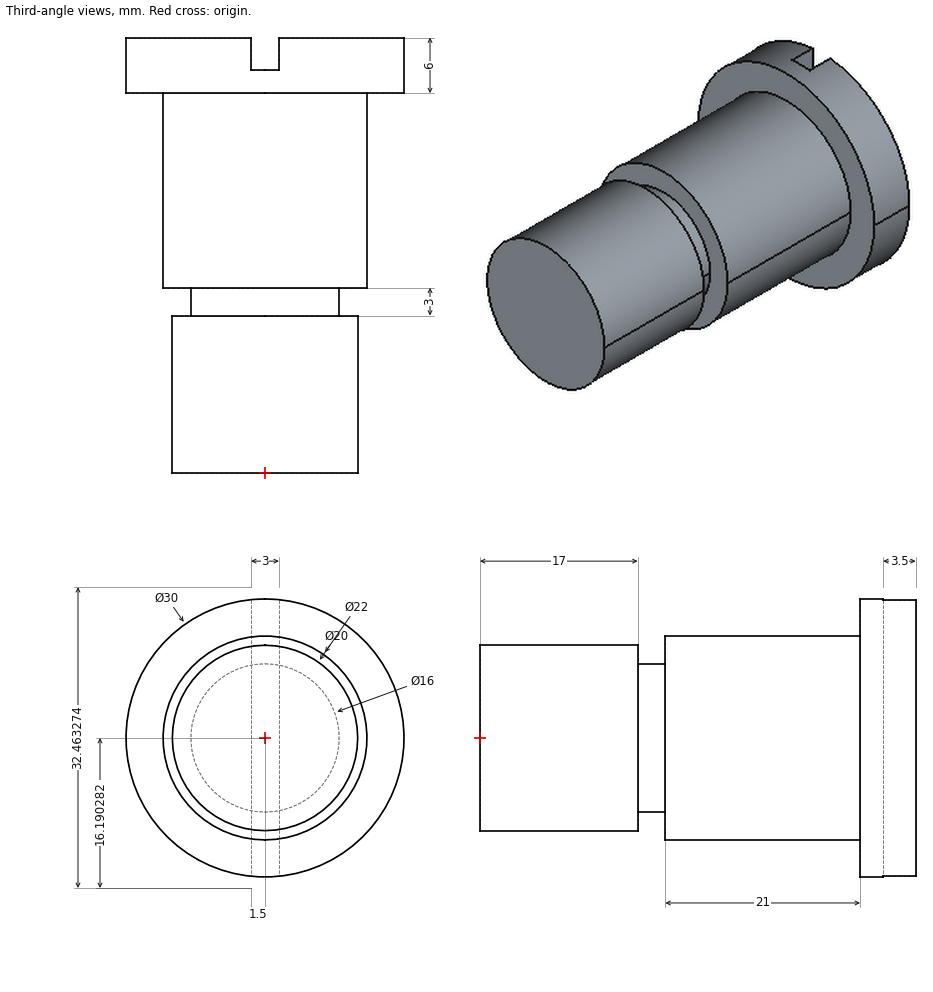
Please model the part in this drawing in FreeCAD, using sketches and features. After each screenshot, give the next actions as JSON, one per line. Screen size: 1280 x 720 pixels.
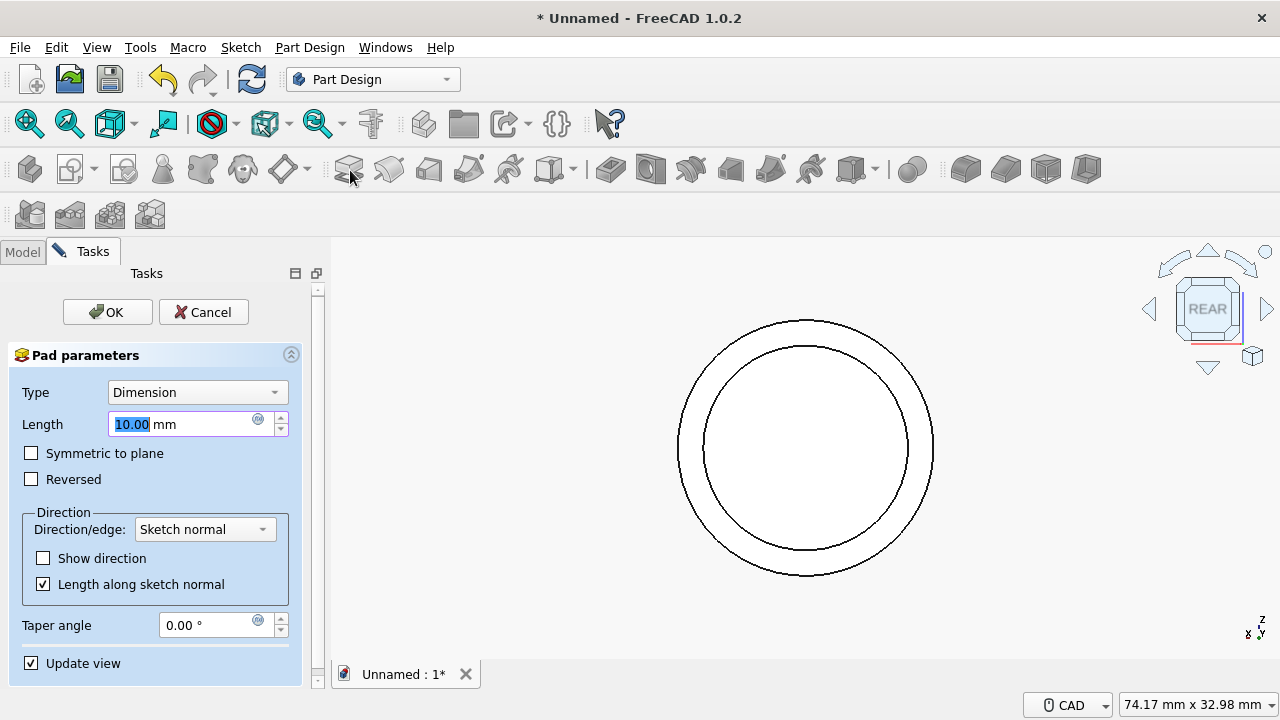
{"action": "type", "text": "3"}
{"action": "key", "text": "Tab"}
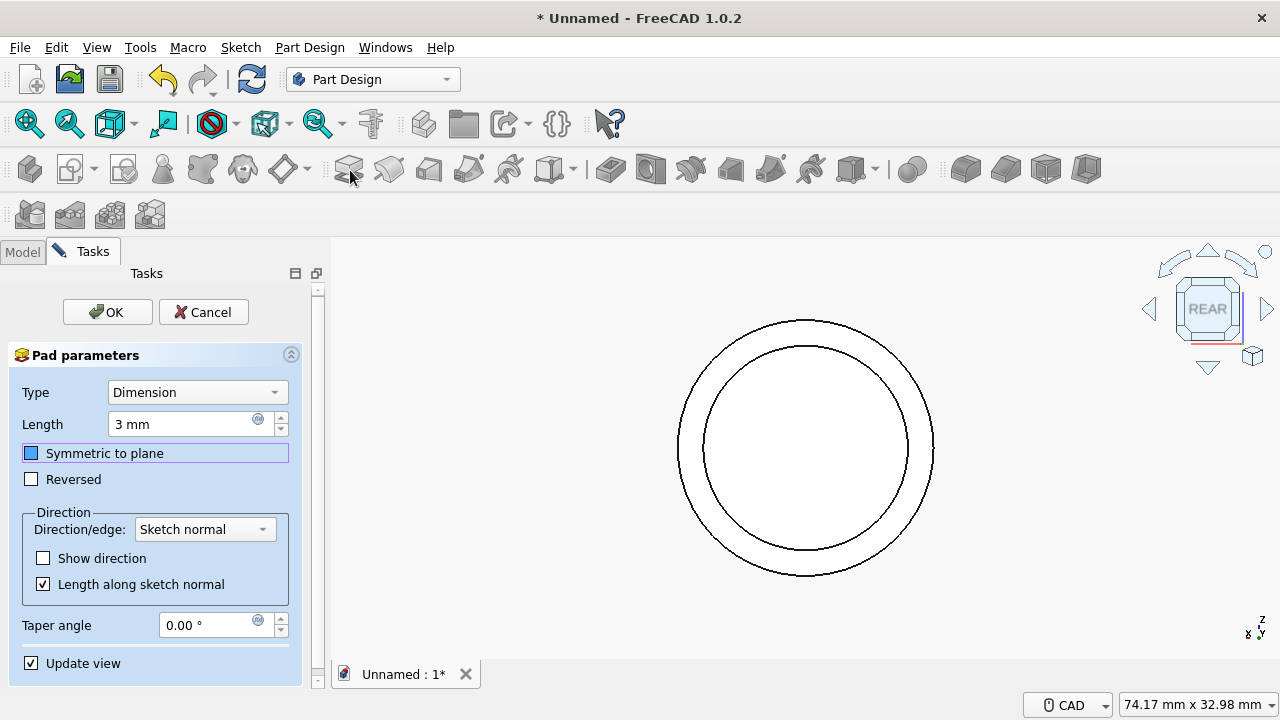
{"action": "left_click", "coordinate": [108, 312]}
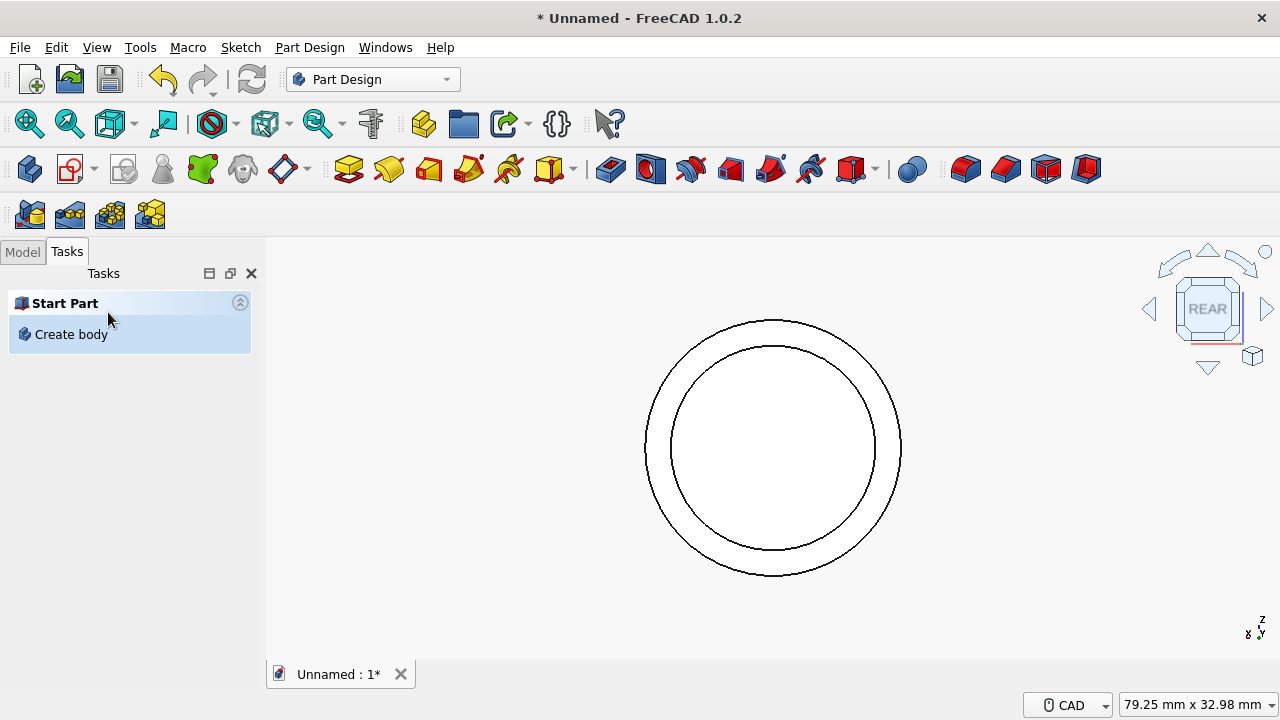
{"action": "left_click", "coordinate": [773, 447]}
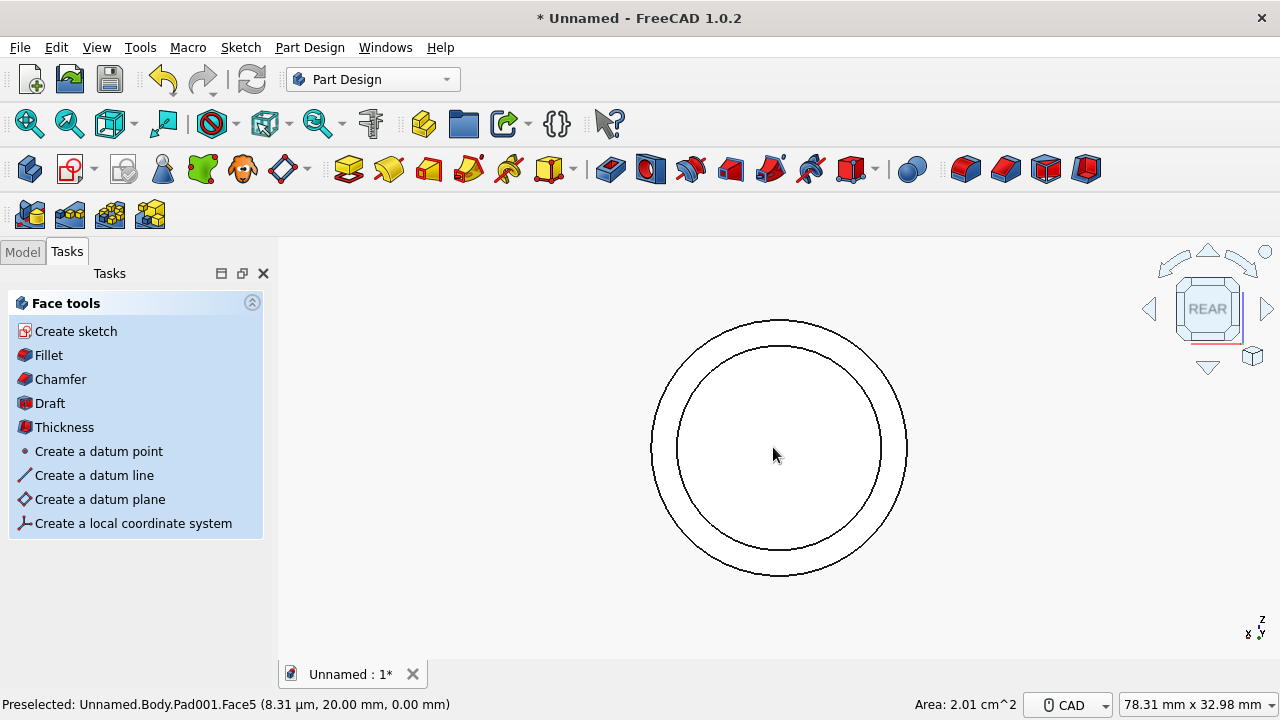
{"action": "left_click", "coordinate": [70, 170]}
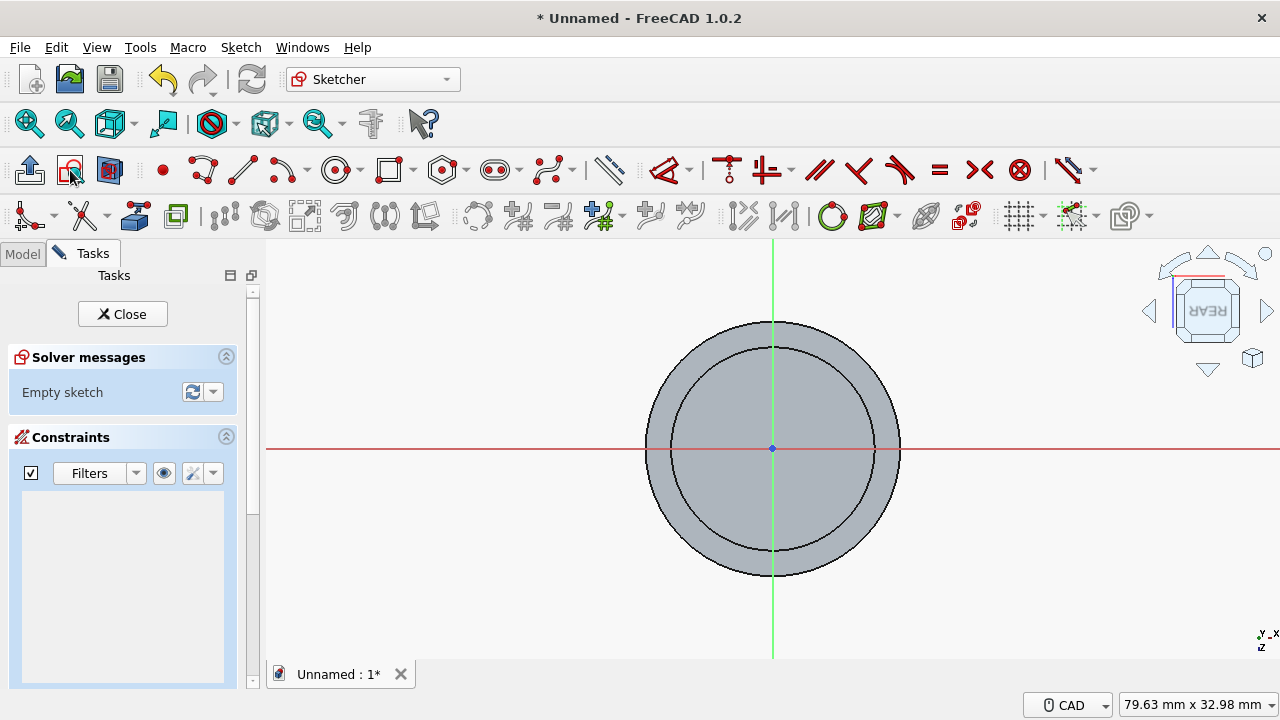
{"action": "left_click", "coordinate": [336, 170]}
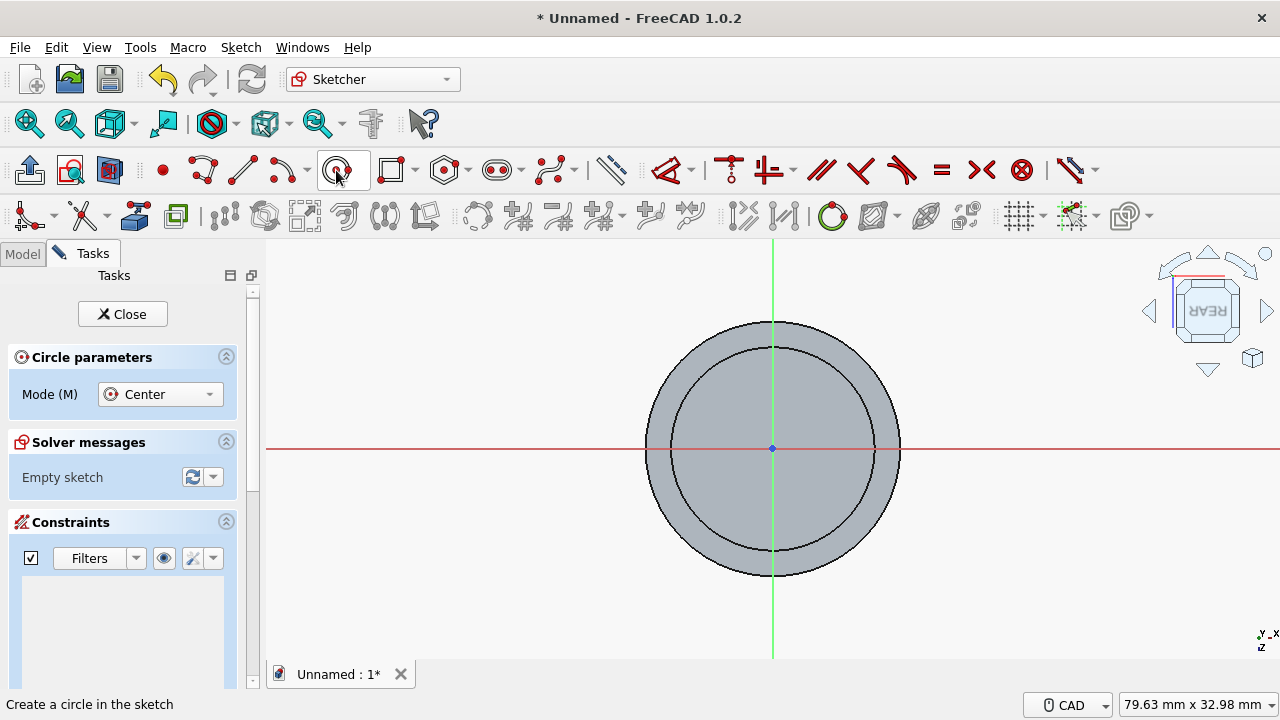
{"action": "left_click", "coordinate": [773, 449]}
{"action": "mouse_move", "coordinate": [872, 350]}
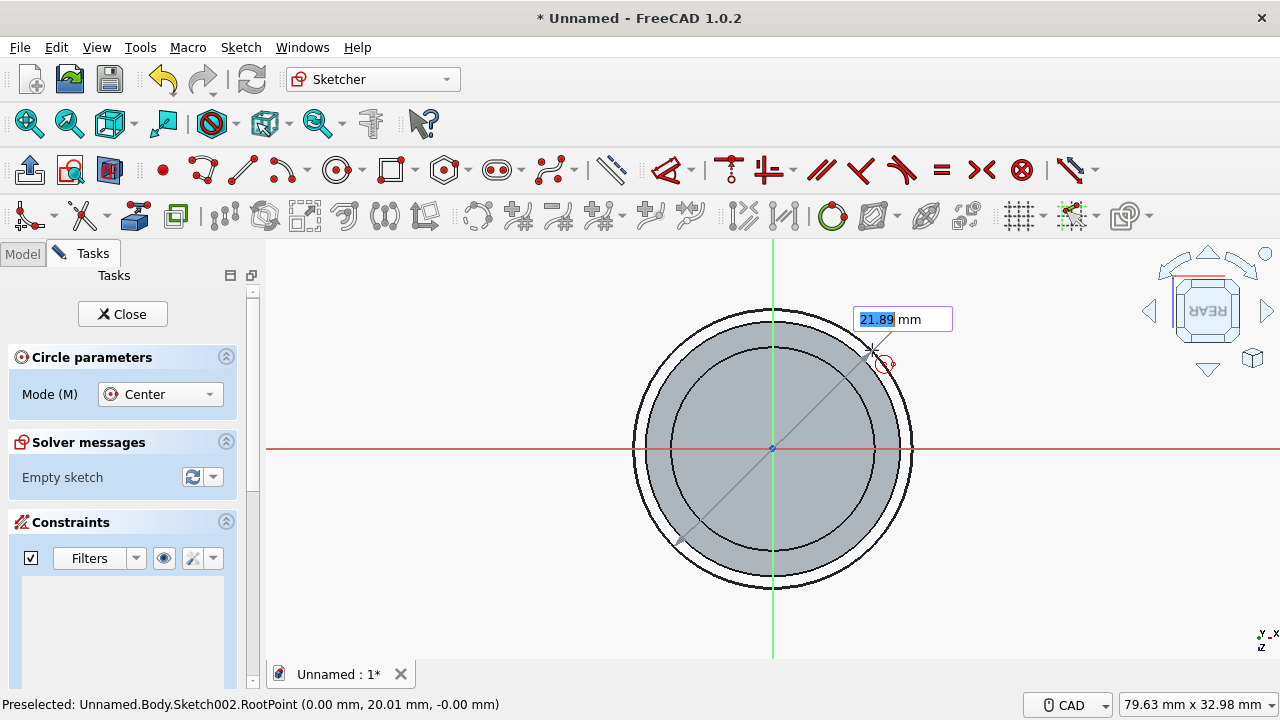
{"action": "type", "text": "22"}
{"action": "key", "text": "Return"}
{"action": "key", "text": "Escape"}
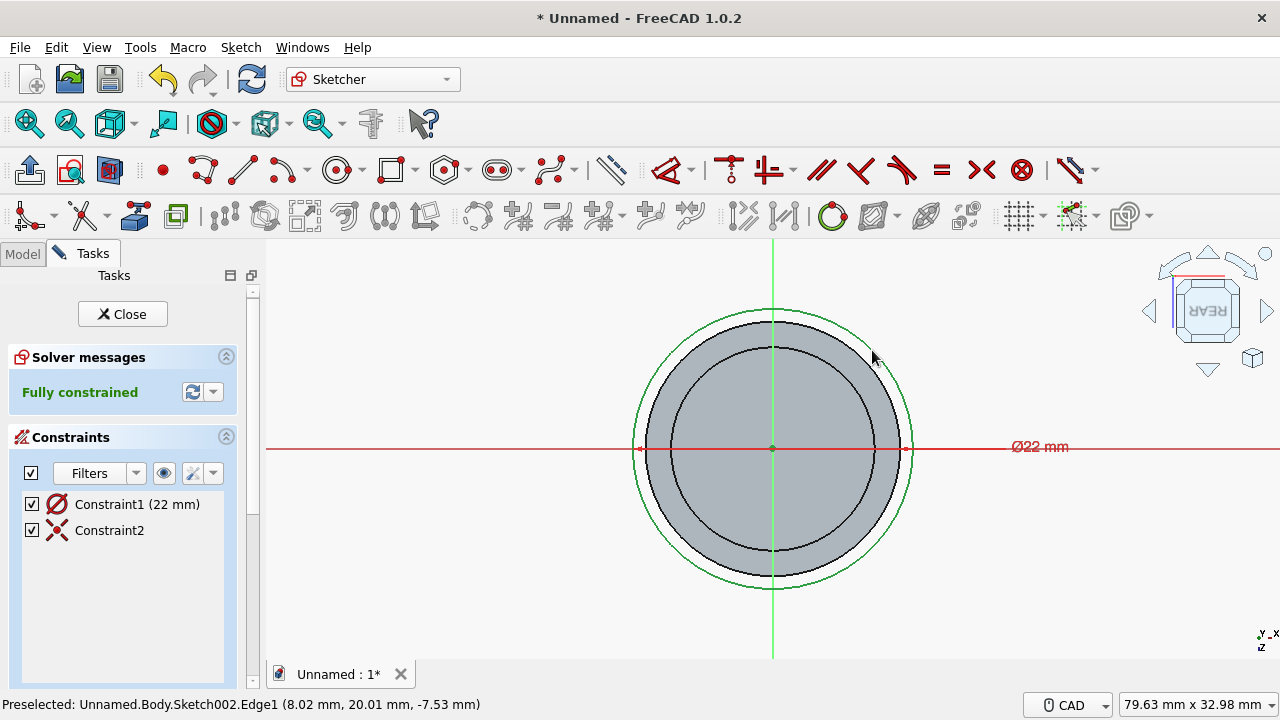
{"action": "left_click", "coordinate": [123, 314]}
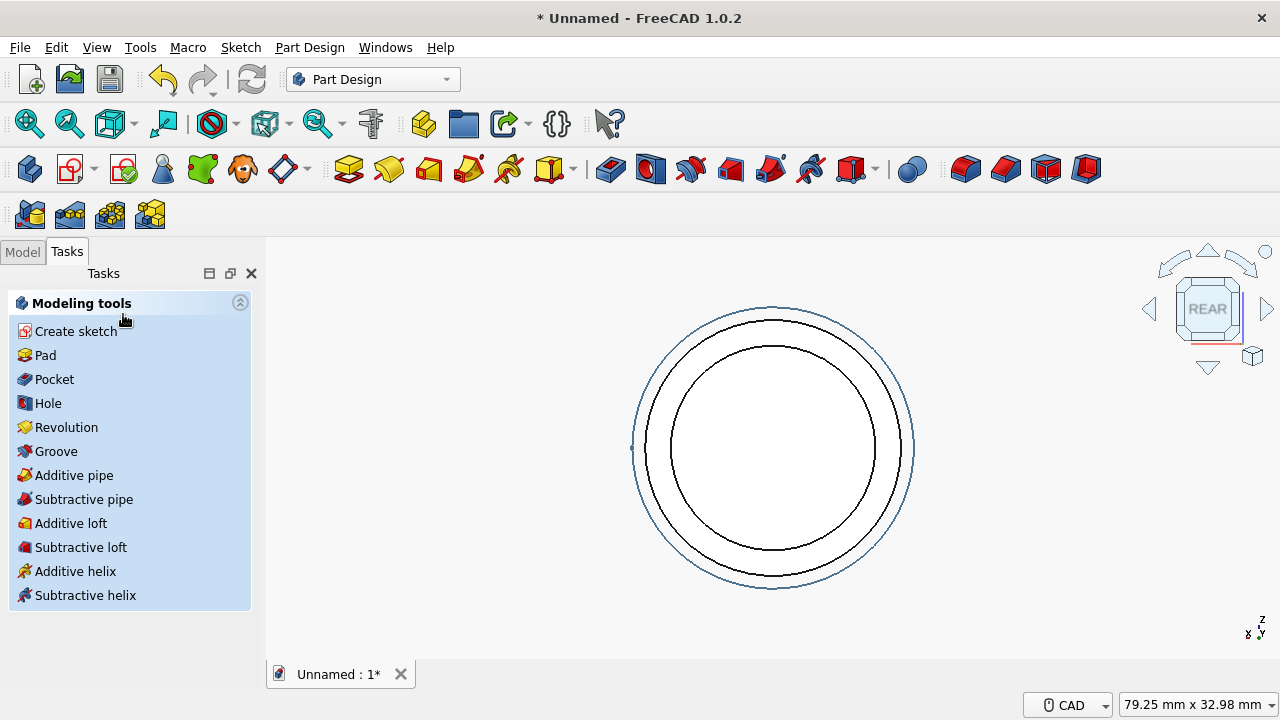
{"action": "left_click", "coordinate": [350, 170]}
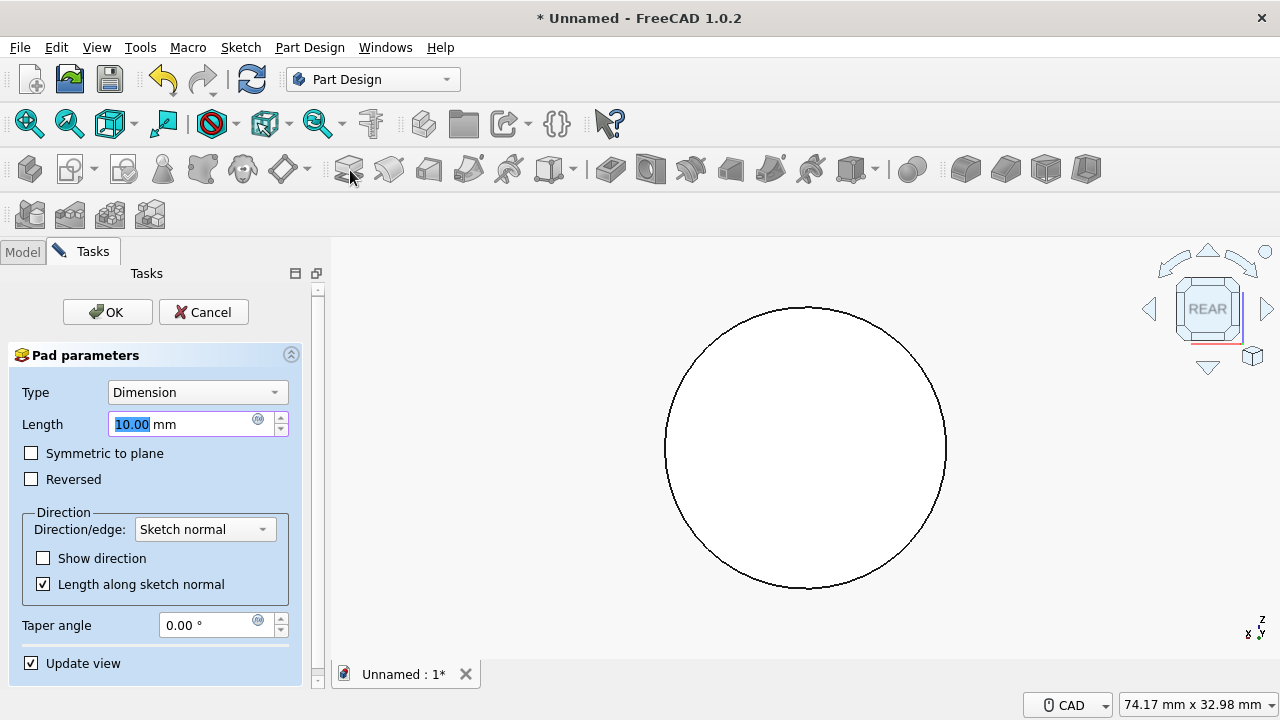
{"action": "type", "text": "21"}
{"action": "key", "text": "Tab"}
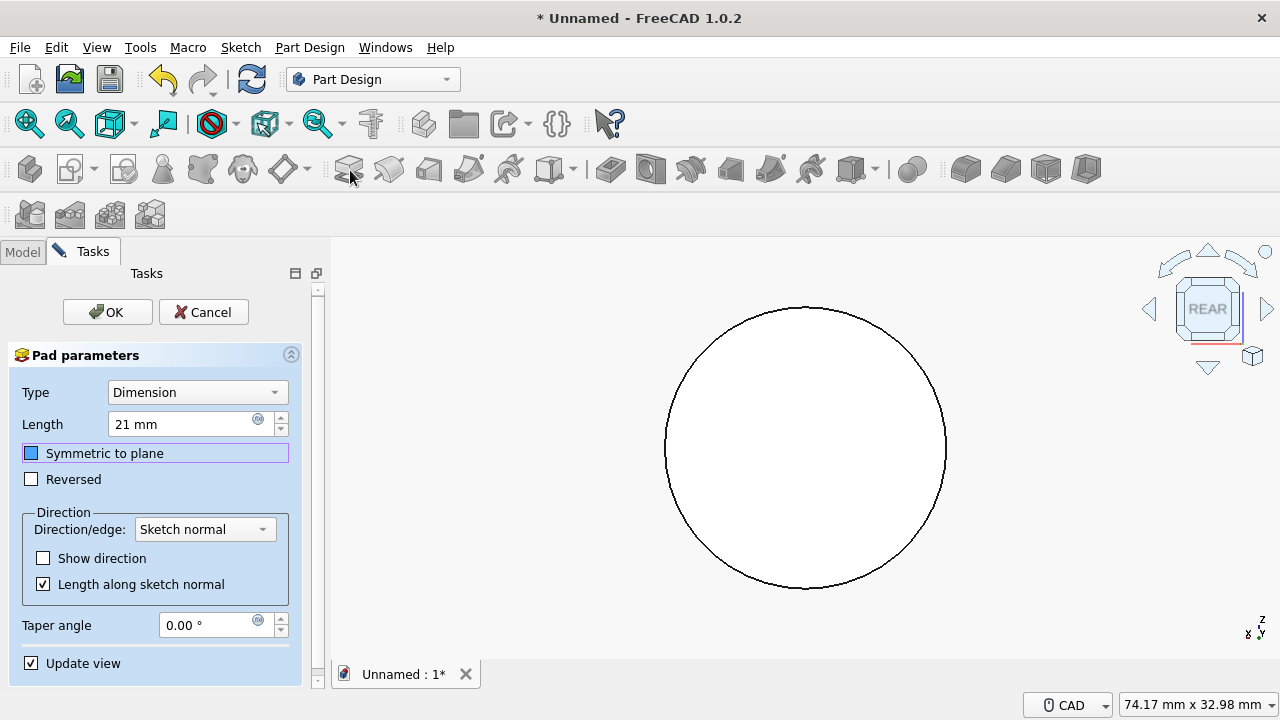
{"action": "left_click", "coordinate": [108, 312]}